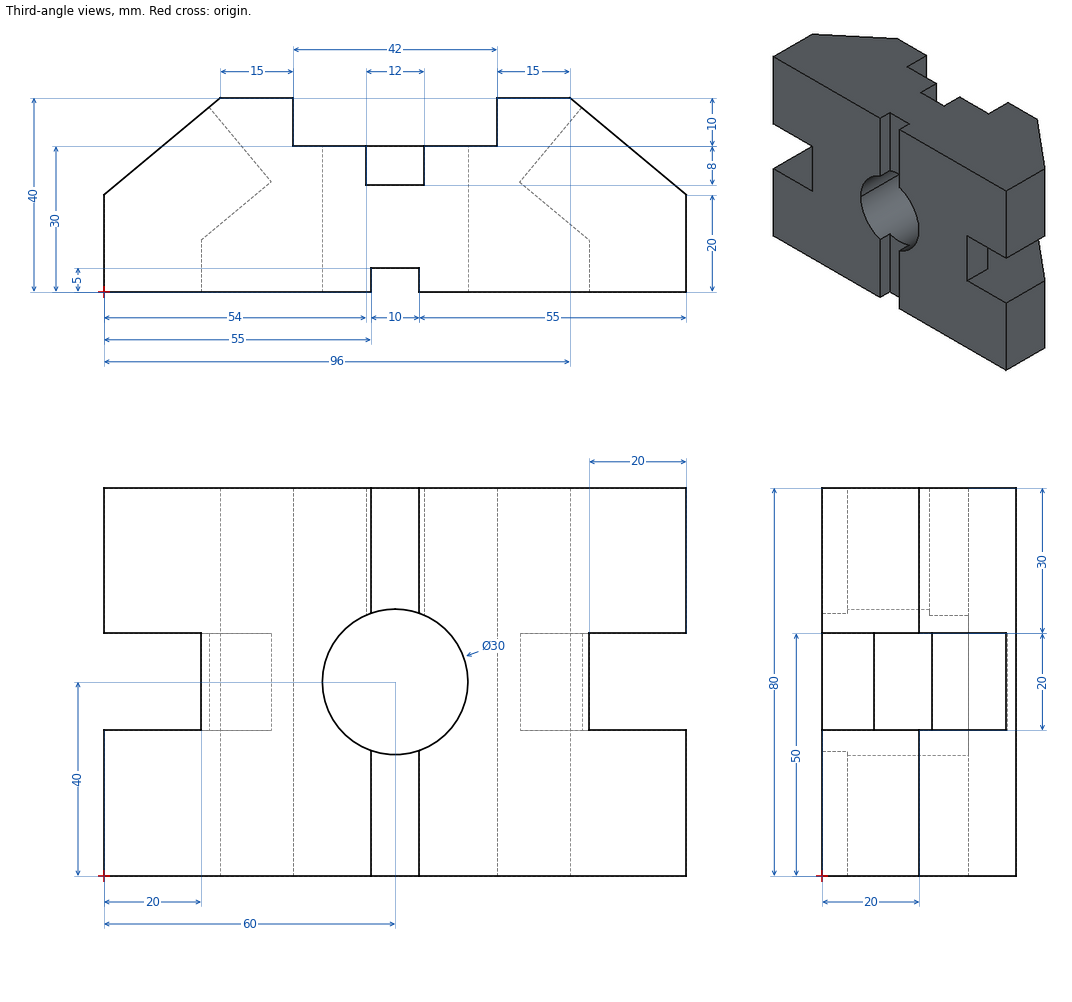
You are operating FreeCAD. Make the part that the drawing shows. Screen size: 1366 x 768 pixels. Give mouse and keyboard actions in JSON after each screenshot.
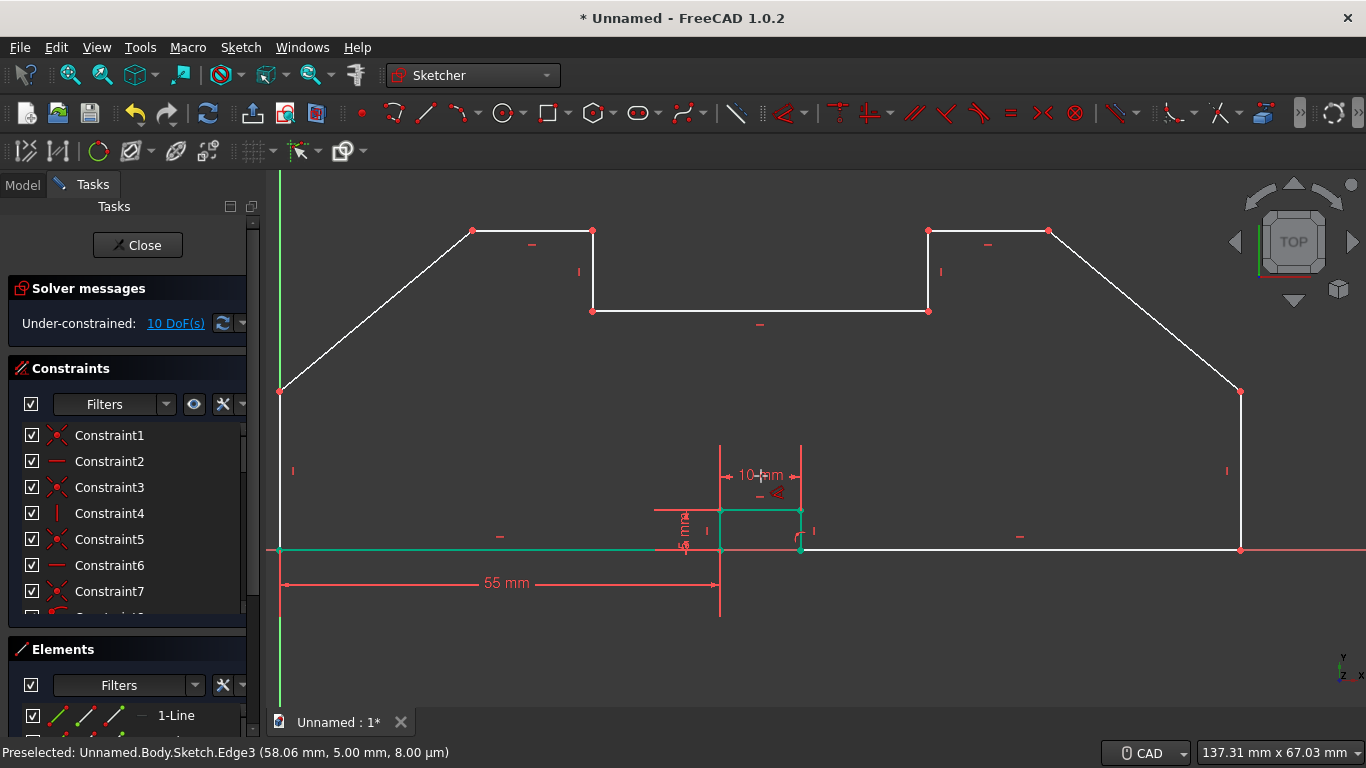
{"action": "left_click", "coordinate": [933, 550]}
{"action": "left_click", "coordinate": [1001, 584]}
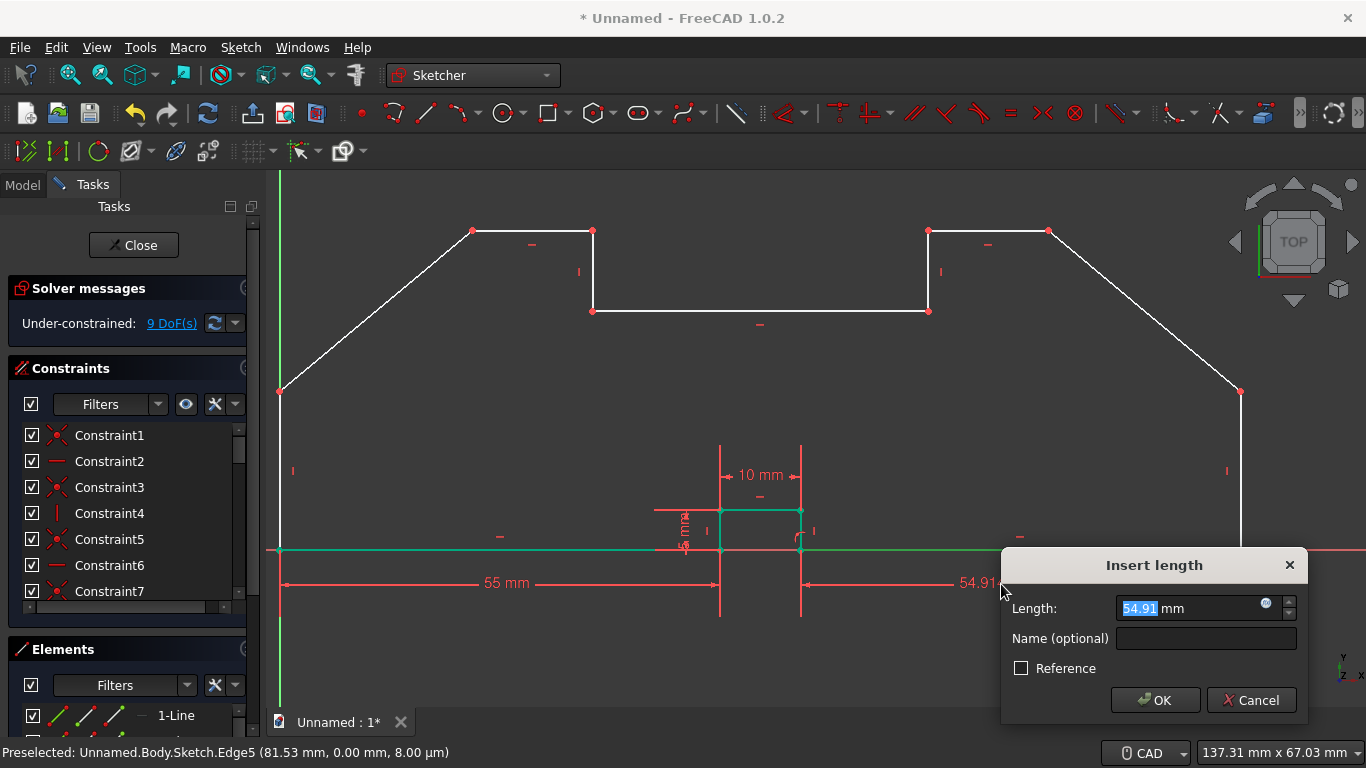
{"action": "type", "text": "55"}
{"action": "key", "text": "Return"}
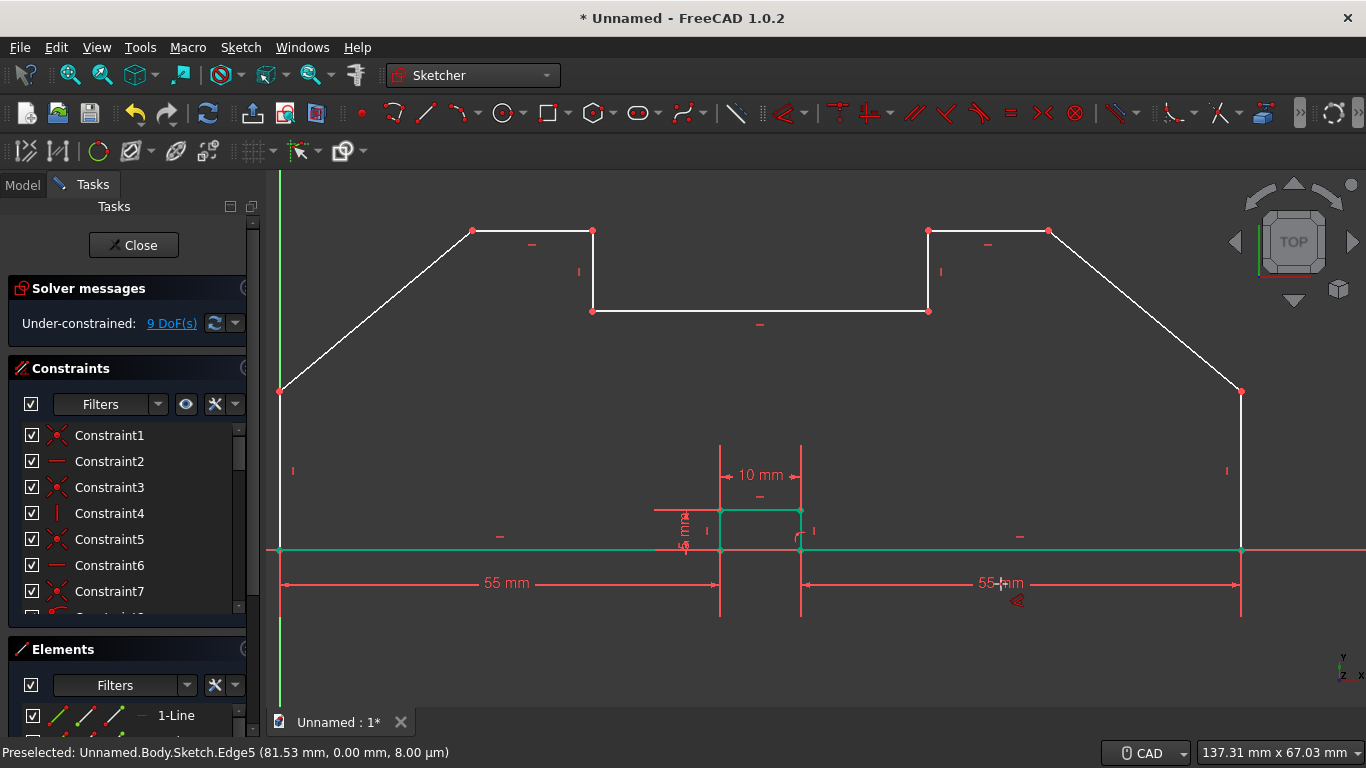
{"action": "scroll", "coordinate": [721, 537], "scroll_direction": "down", "scroll_amount": 2}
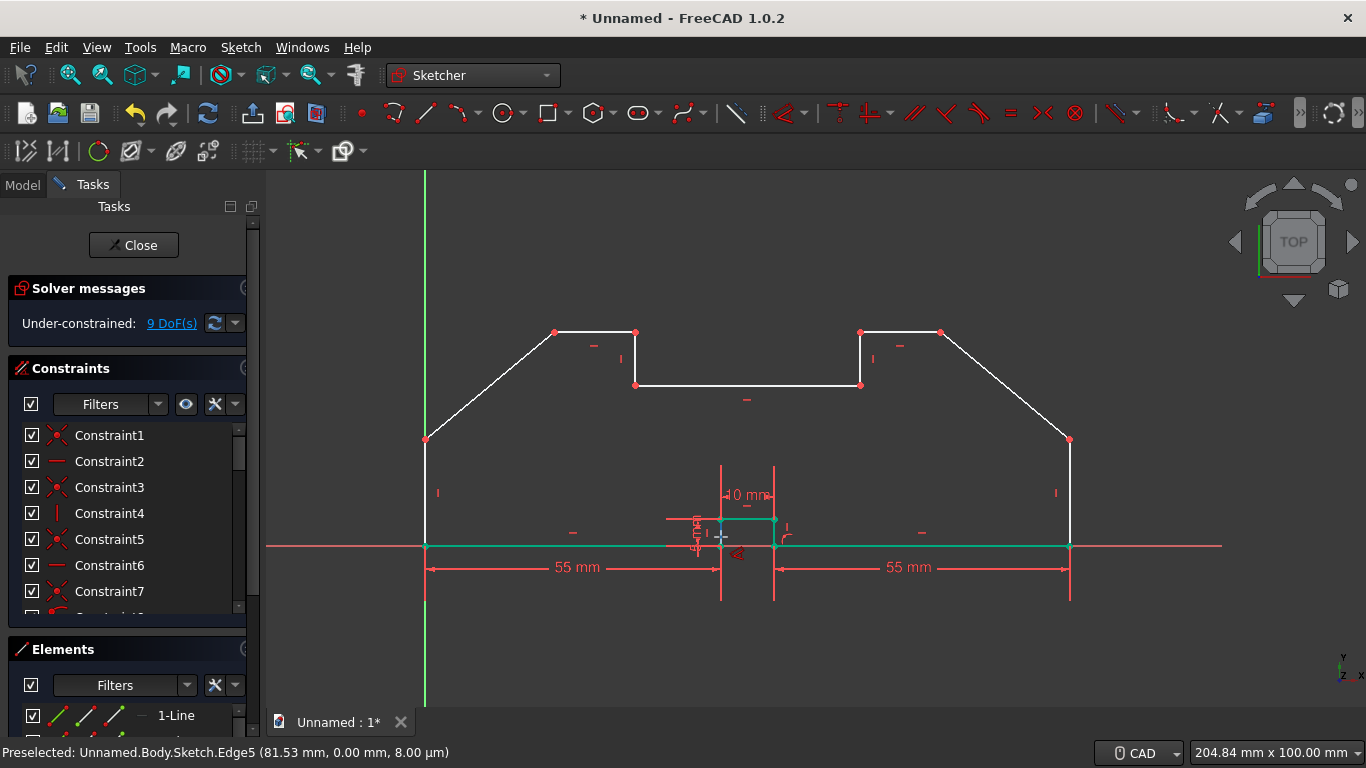
{"action": "left_click", "coordinate": [1070, 514]}
{"action": "left_click", "coordinate": [1104, 493]}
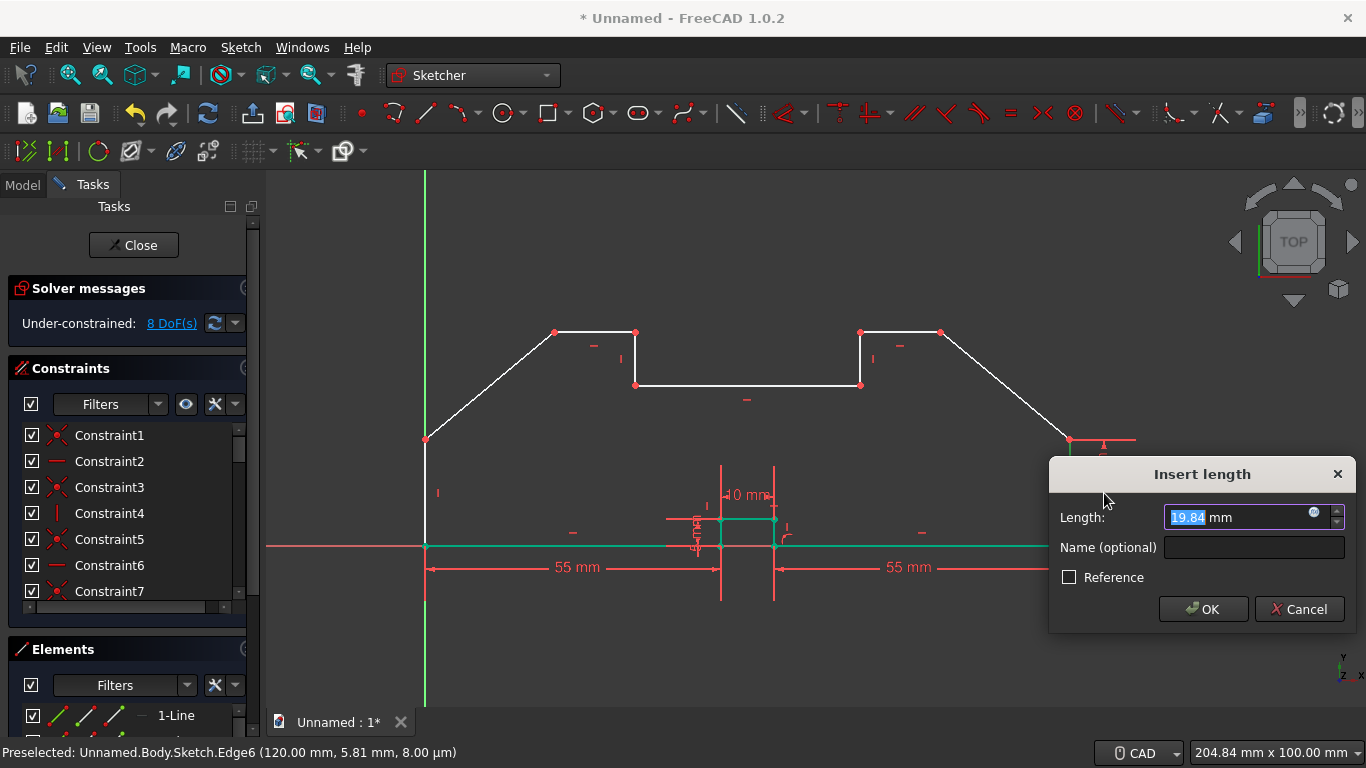
{"action": "type", "text": "20"}
{"action": "key", "text": "Return"}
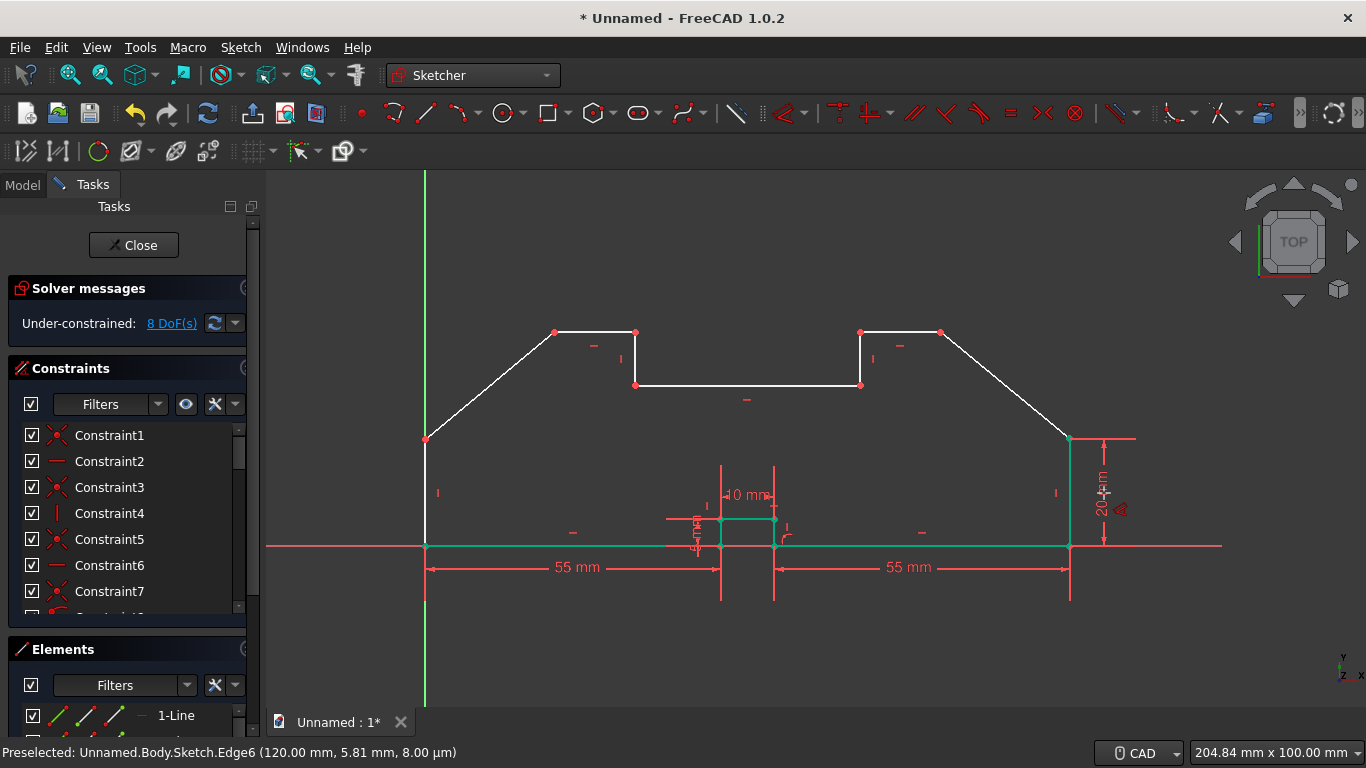
{"action": "left_click", "coordinate": [917, 332]}
{"action": "left_click", "coordinate": [901, 298]}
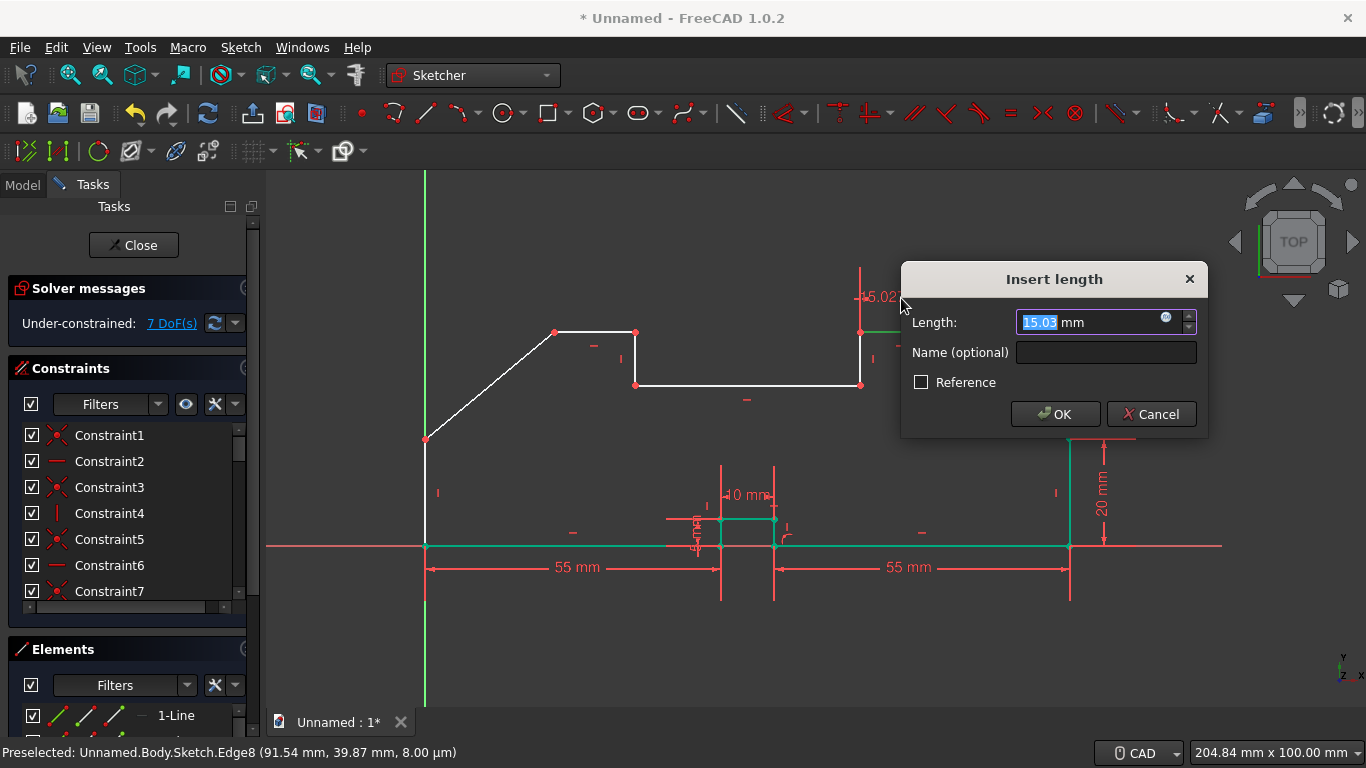
{"action": "type", "text": "15"}
{"action": "key", "text": "Return"}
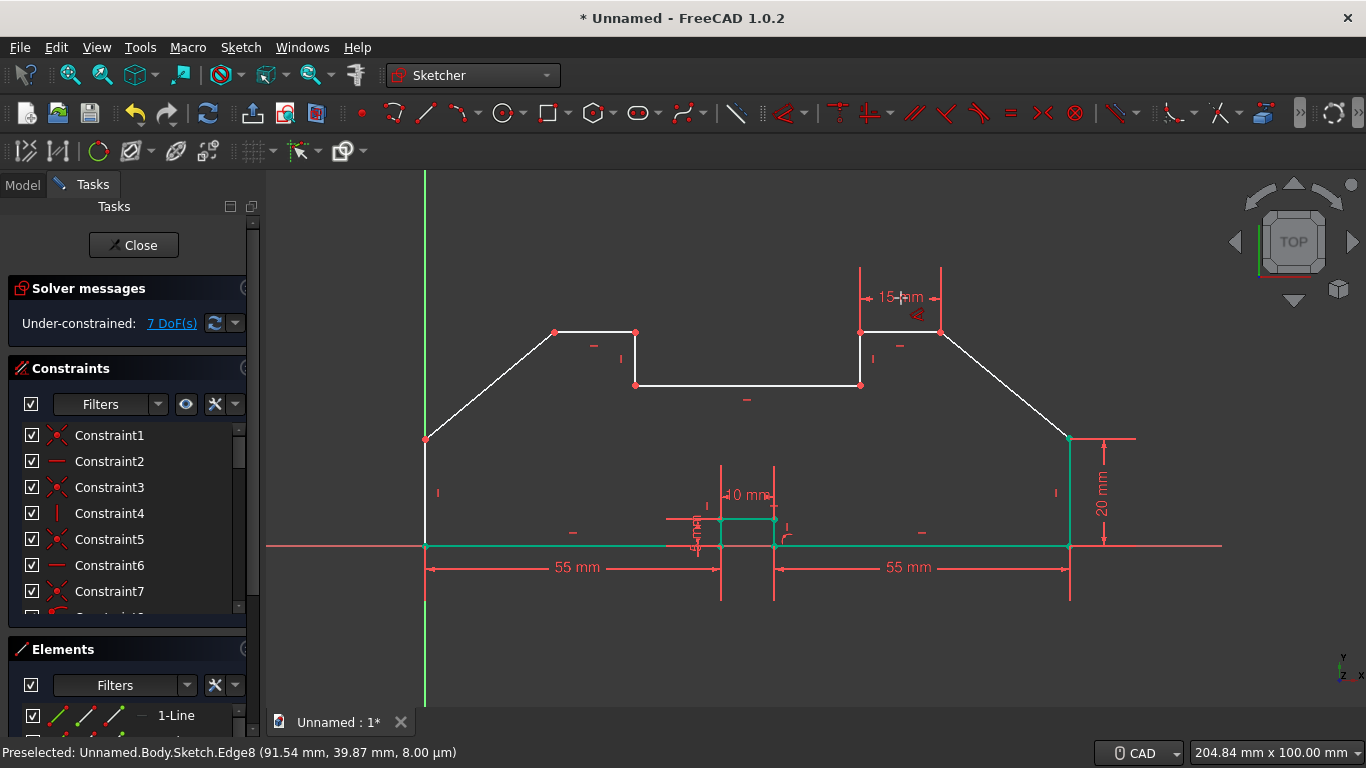
{"action": "left_click", "coordinate": [860, 348]}
{"action": "left_click", "coordinate": [894, 359]}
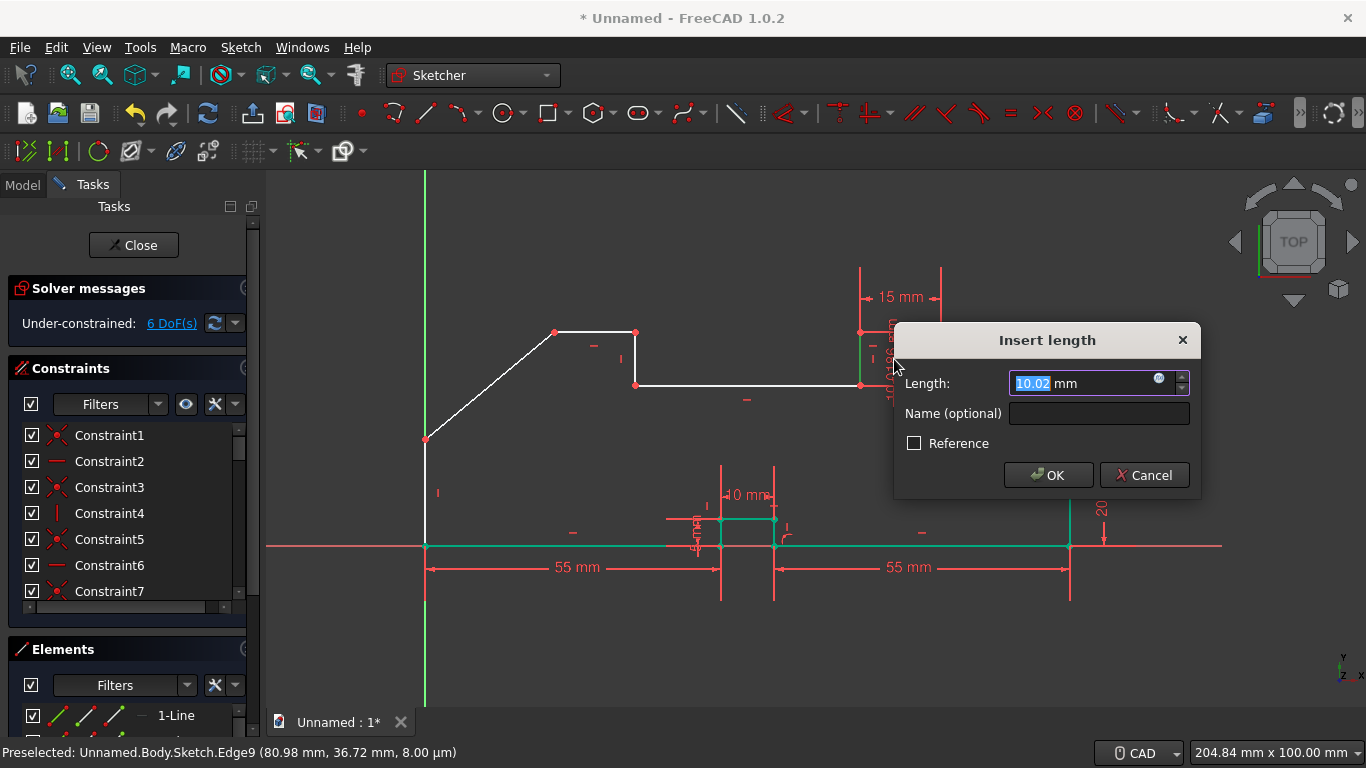
{"action": "type", "text": "10"}
{"action": "key", "text": "Return"}